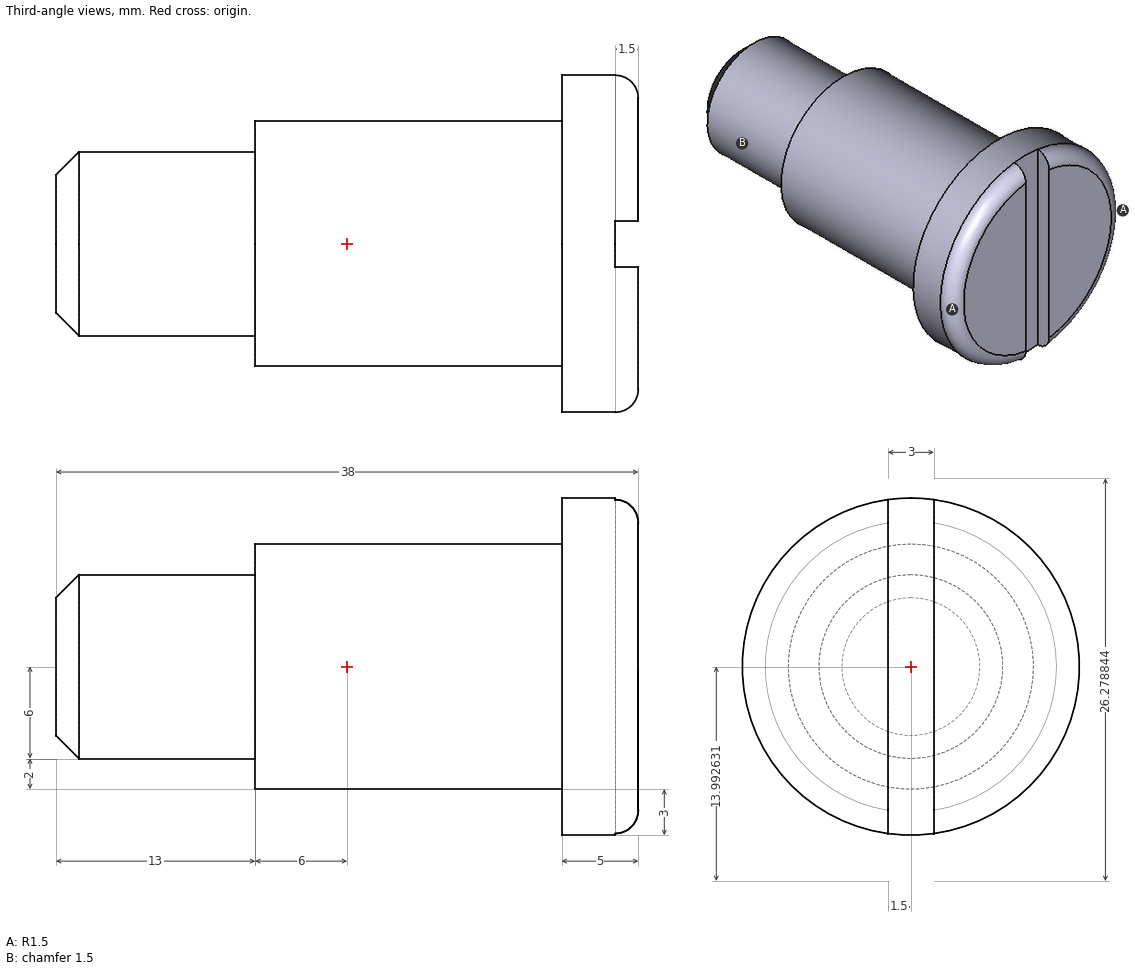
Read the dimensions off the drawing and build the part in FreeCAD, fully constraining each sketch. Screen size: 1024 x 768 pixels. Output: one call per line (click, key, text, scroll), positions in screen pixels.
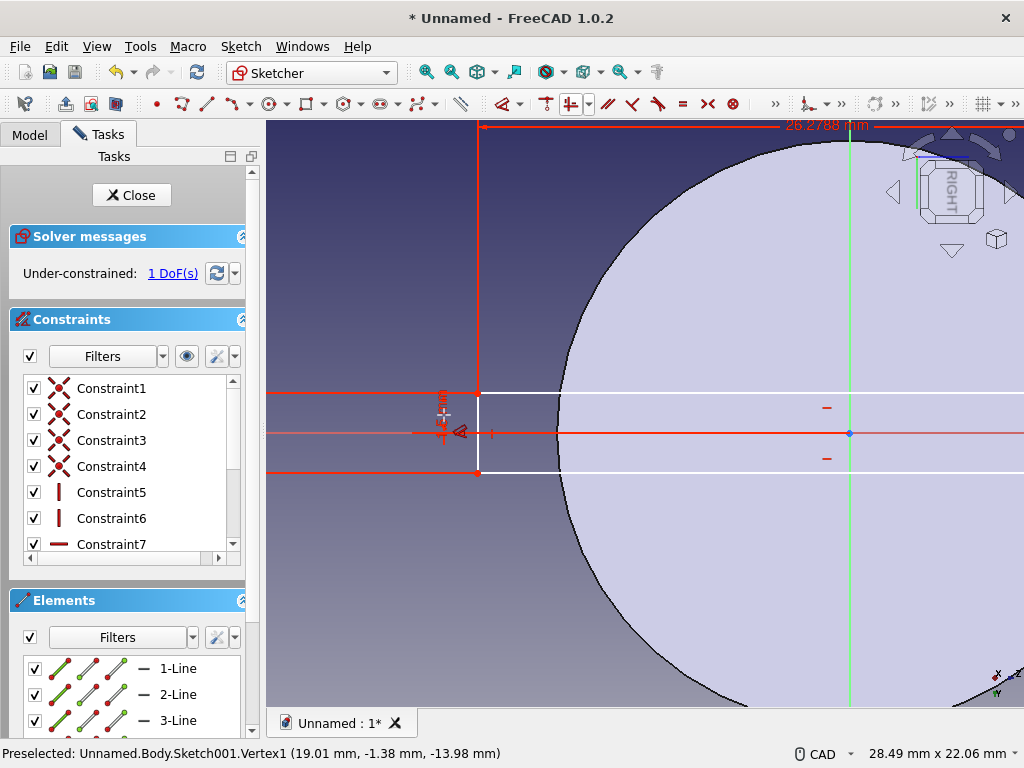
click(478, 393)
click(664, 359)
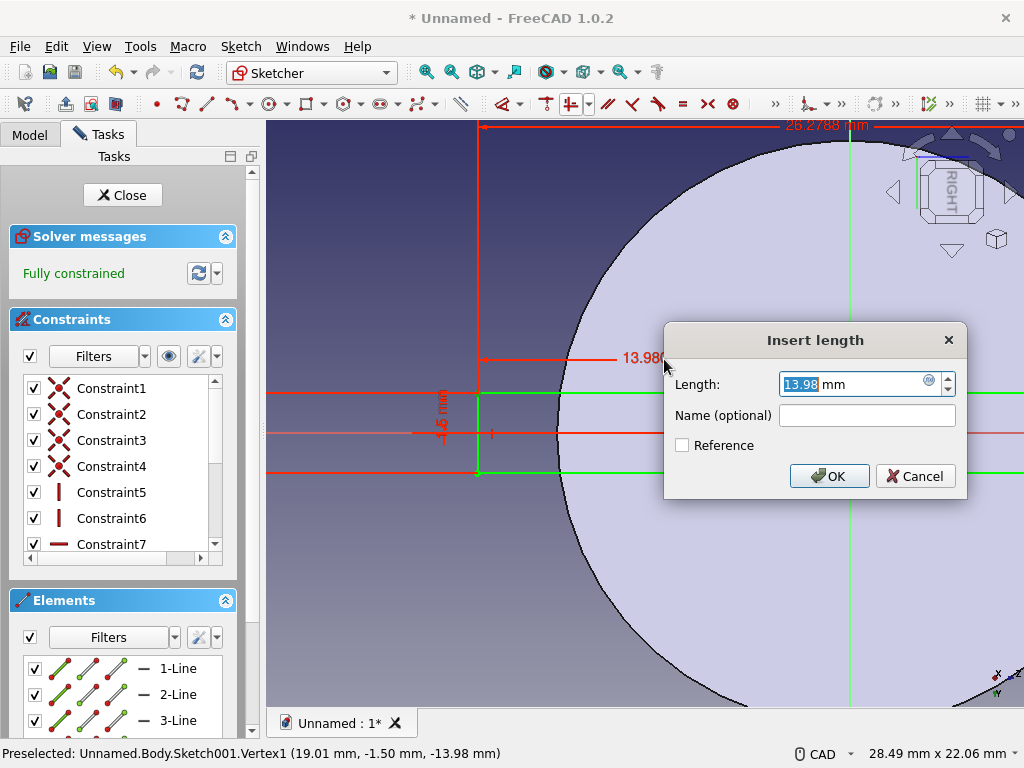
text(13.992631)
key(Return)
key(Escape)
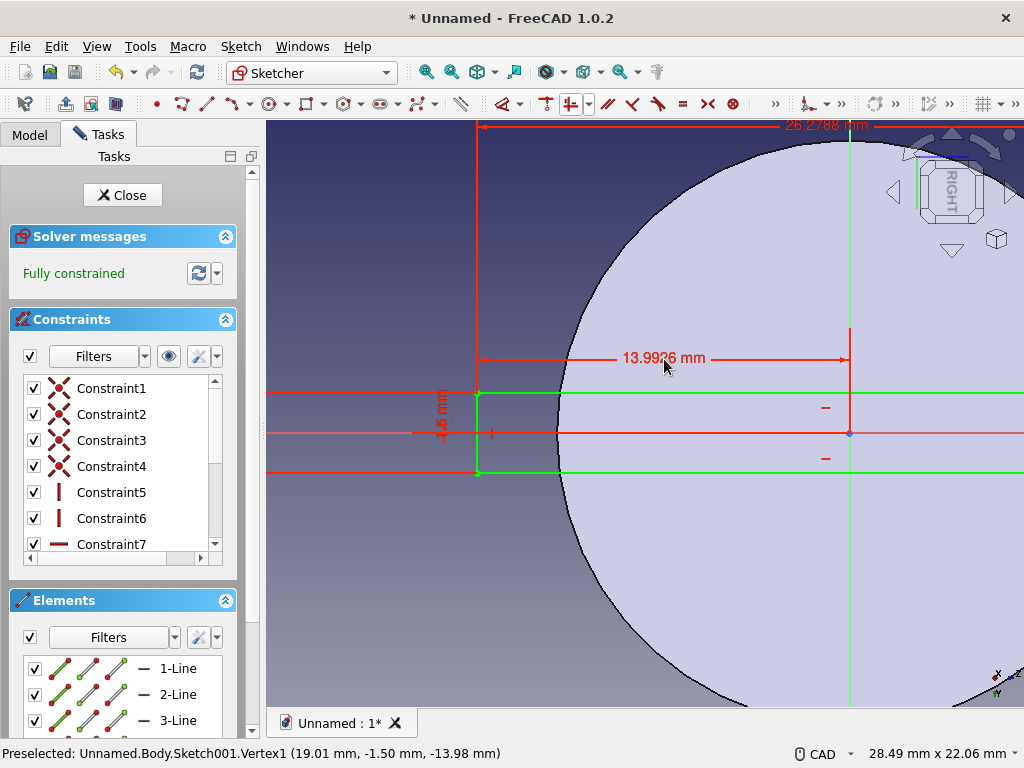
click(123, 195)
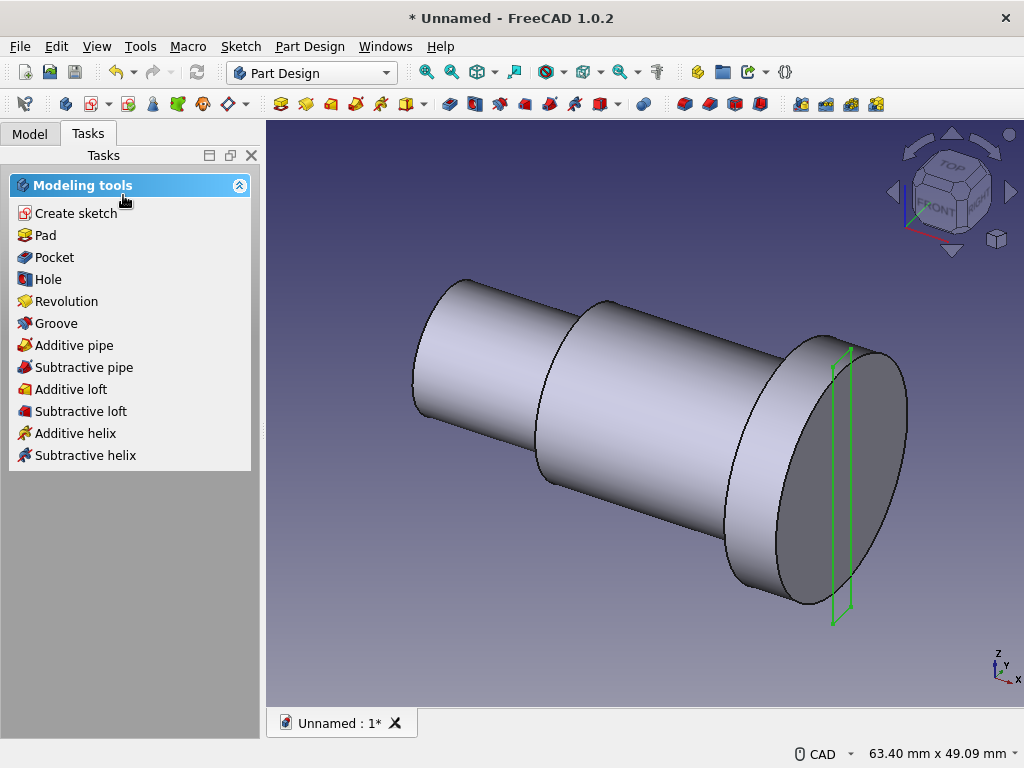
click(450, 104)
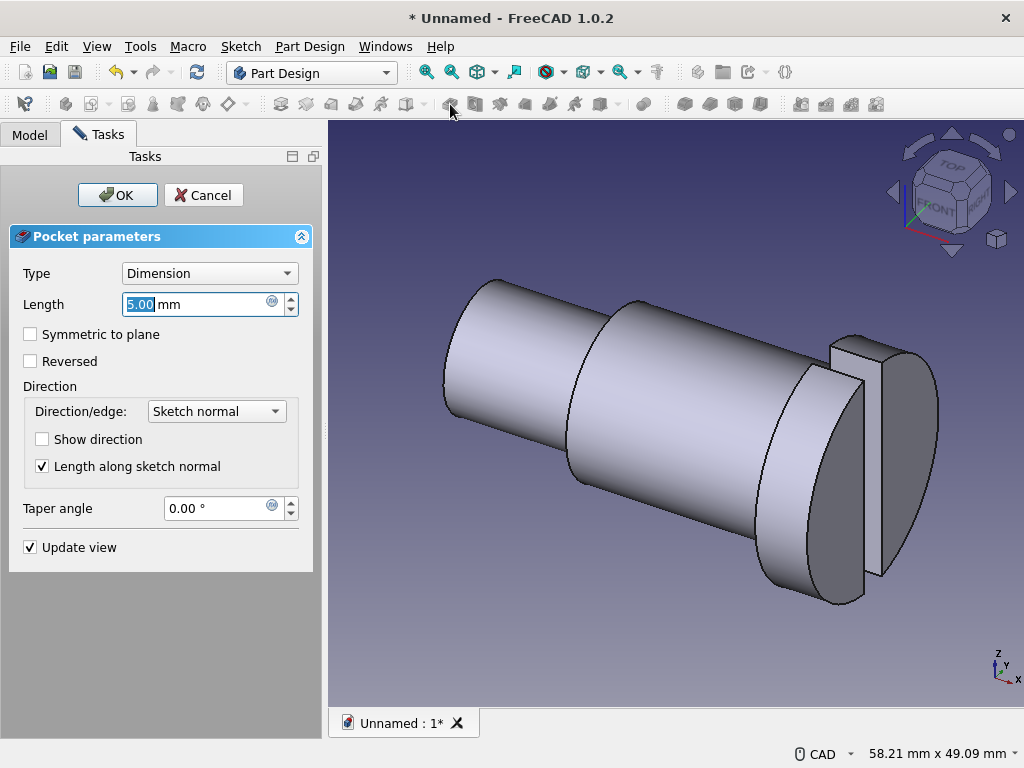
text(1.5)
key(Tab)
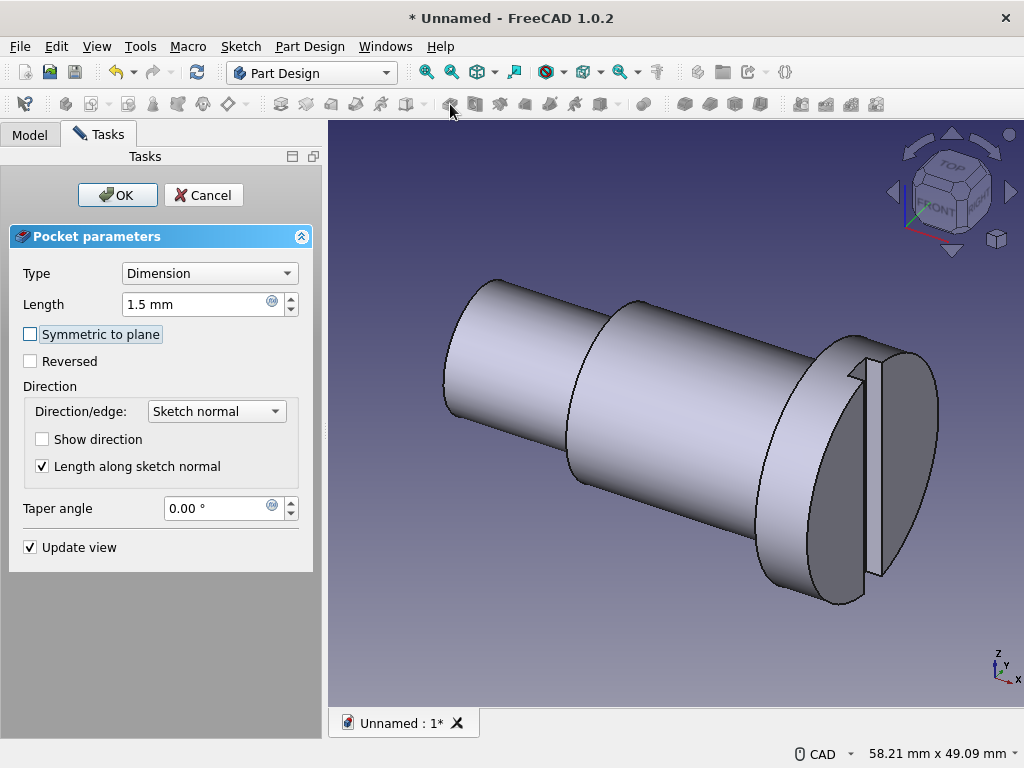
click(118, 195)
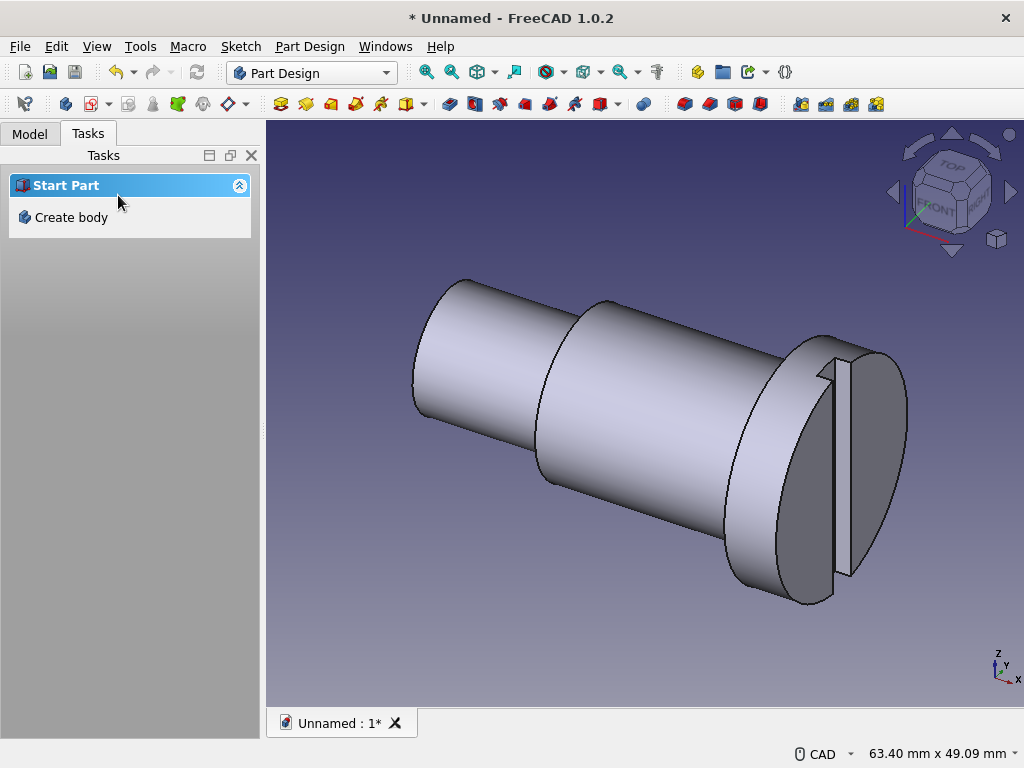
click(776, 543)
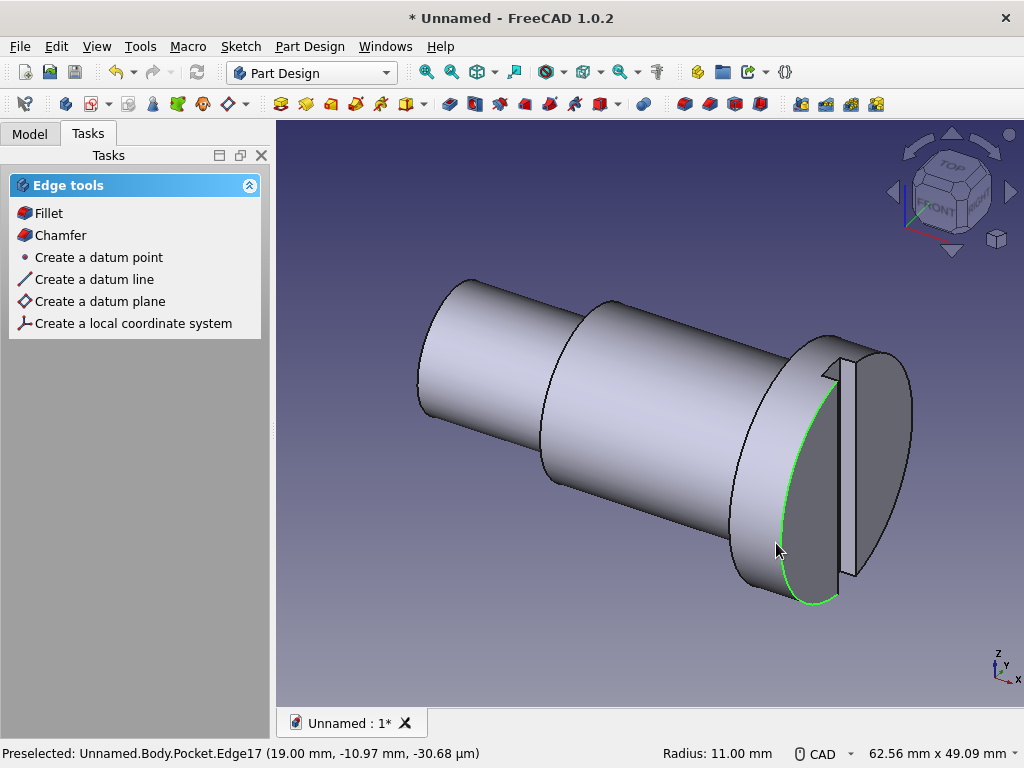
click(890, 353, ctrl)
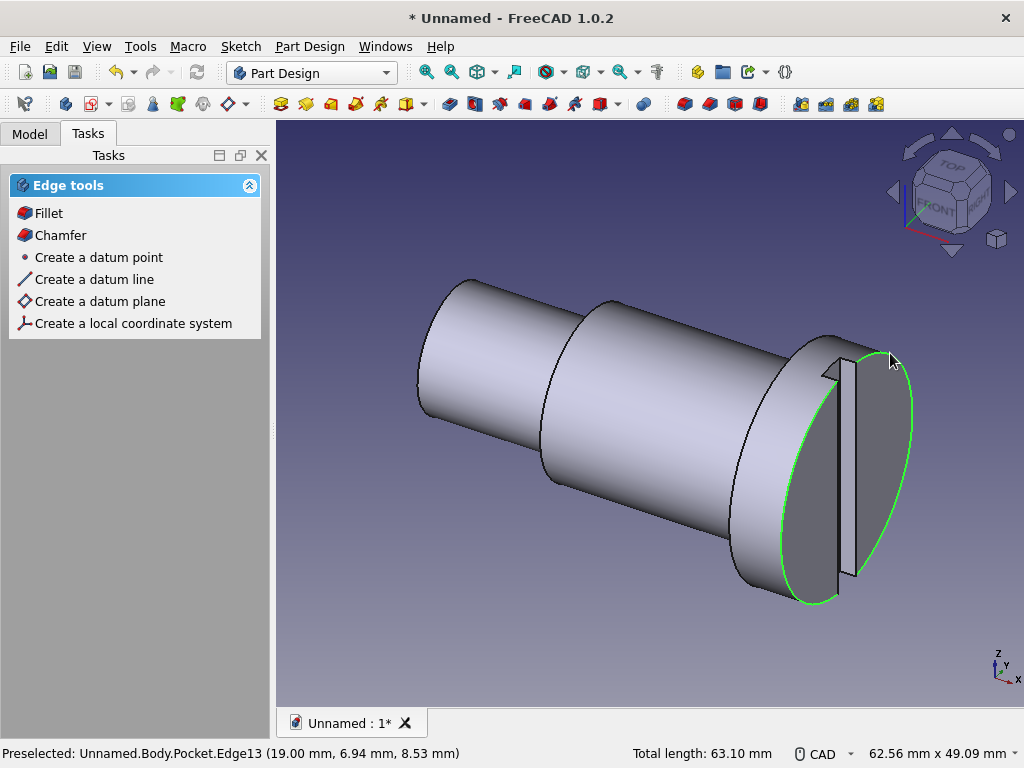
click(685, 104)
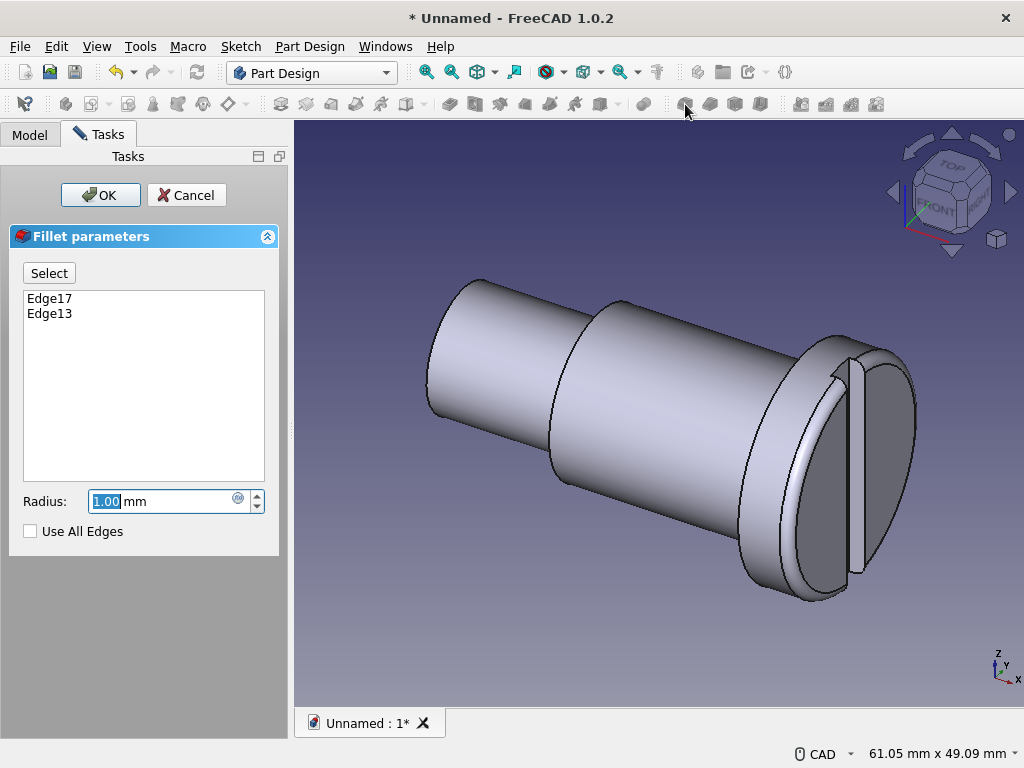
text(1.5)
key(Tab)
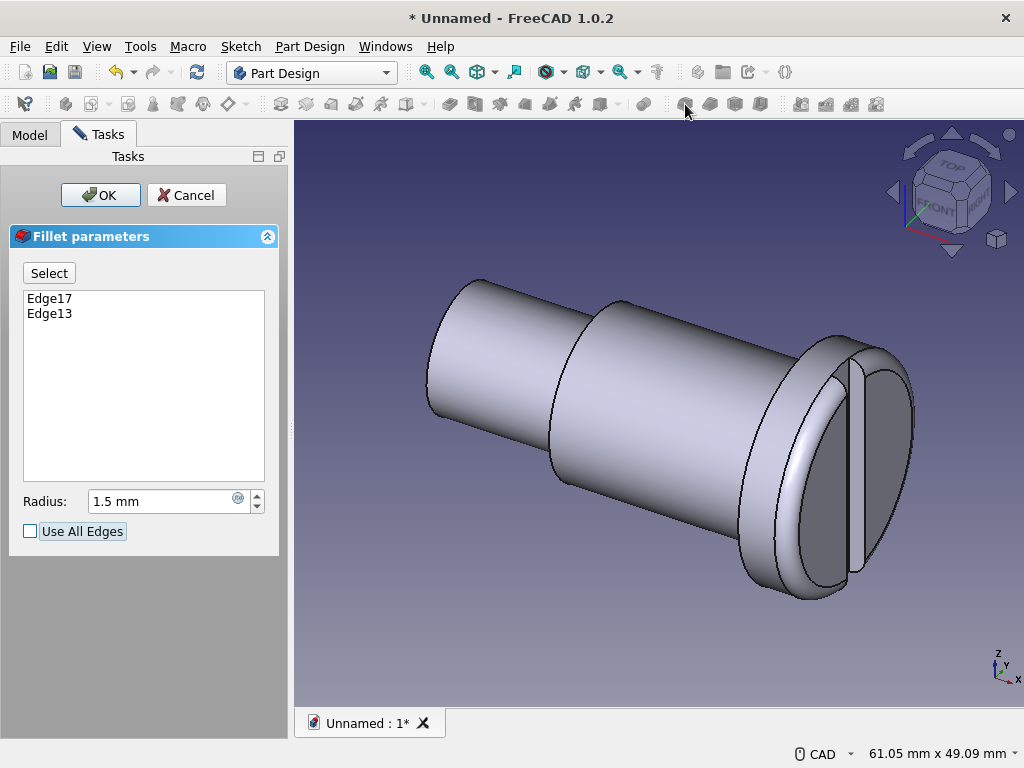
click(101, 195)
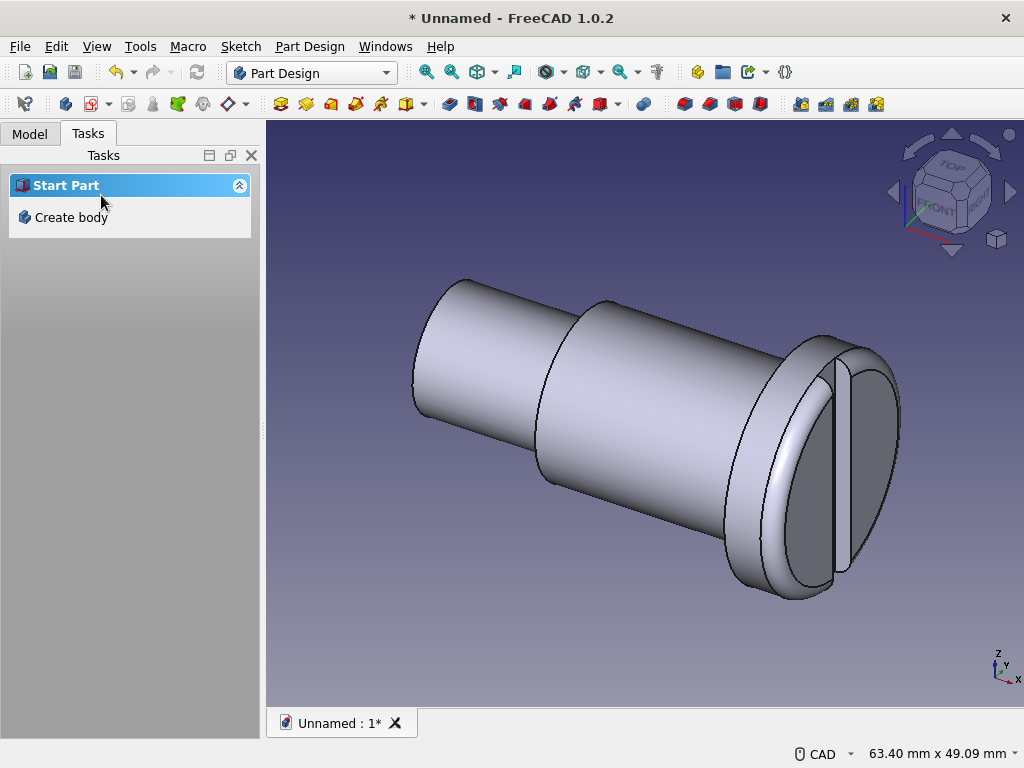
key(0)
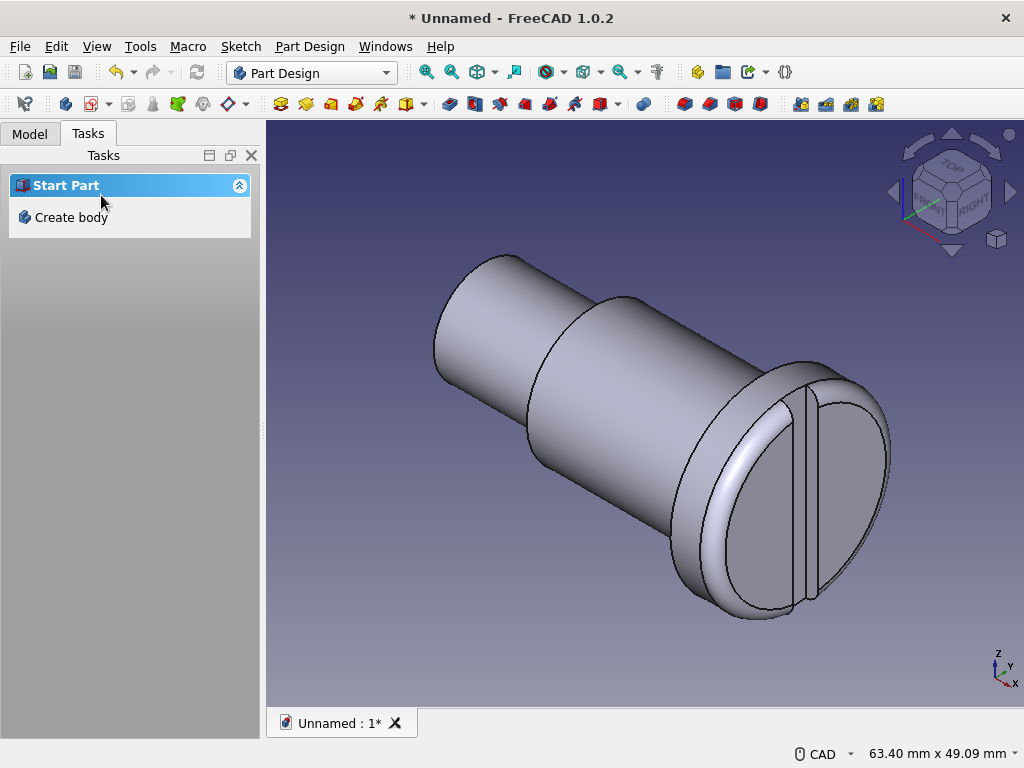
key(2)